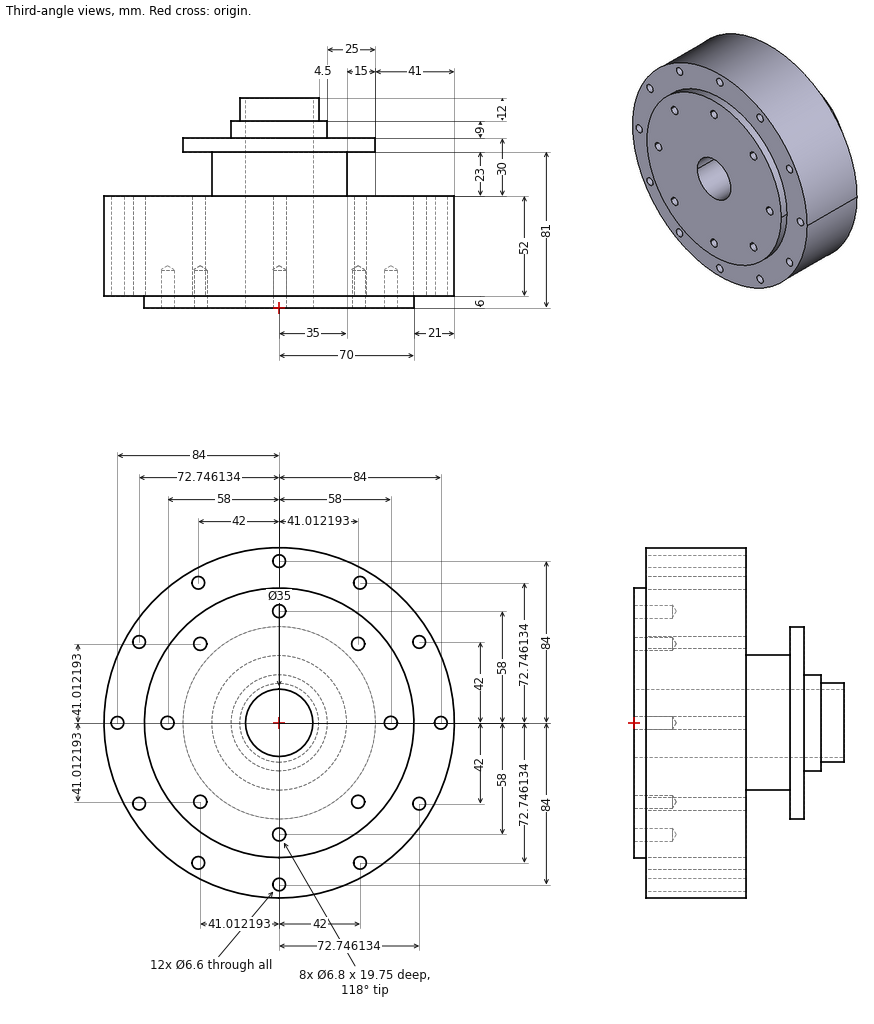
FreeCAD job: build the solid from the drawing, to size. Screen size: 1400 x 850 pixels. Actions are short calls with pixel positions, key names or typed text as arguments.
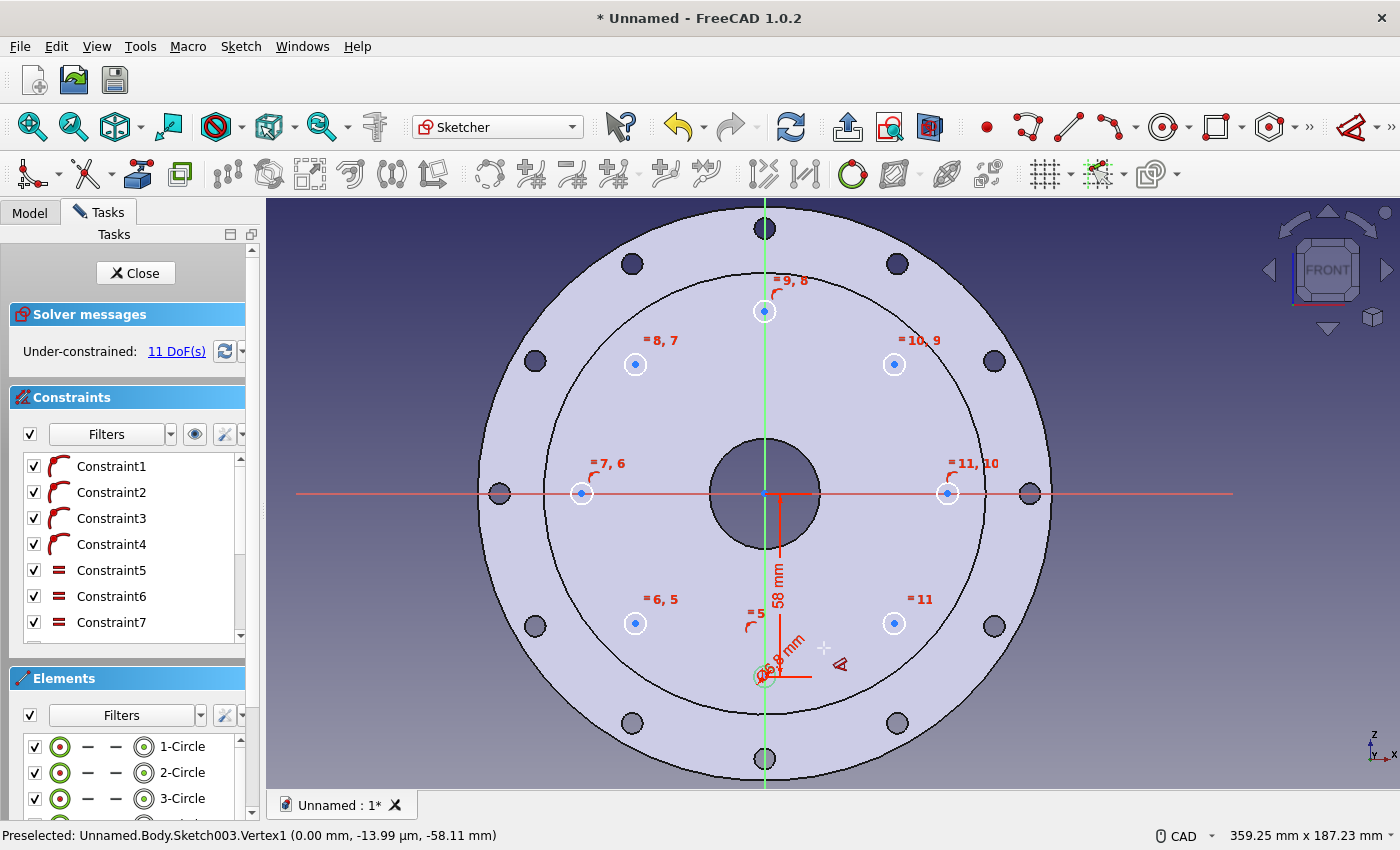
click(582, 494)
click(673, 528)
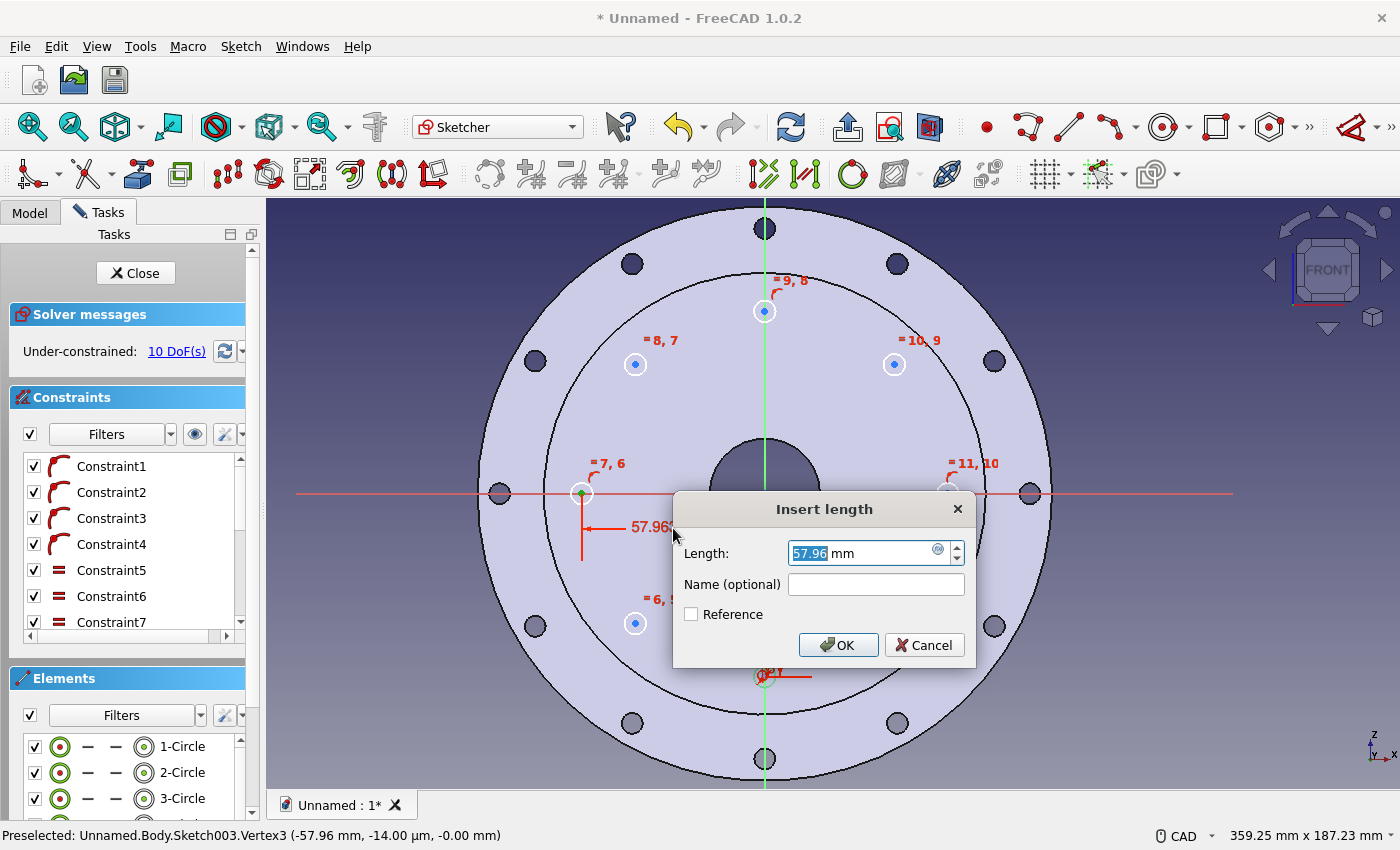
text(58)
key(Return)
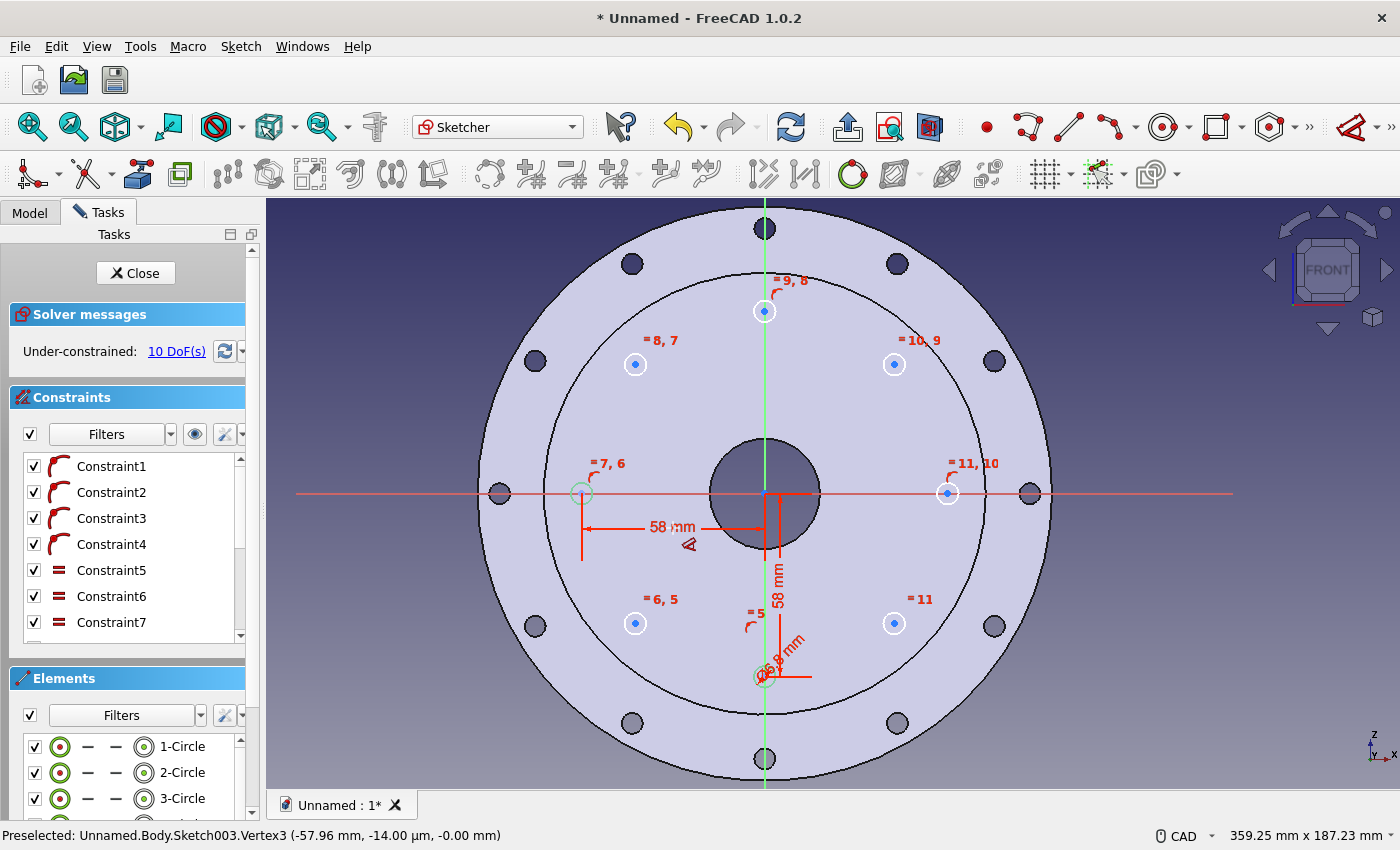
click(765, 311)
click(799, 403)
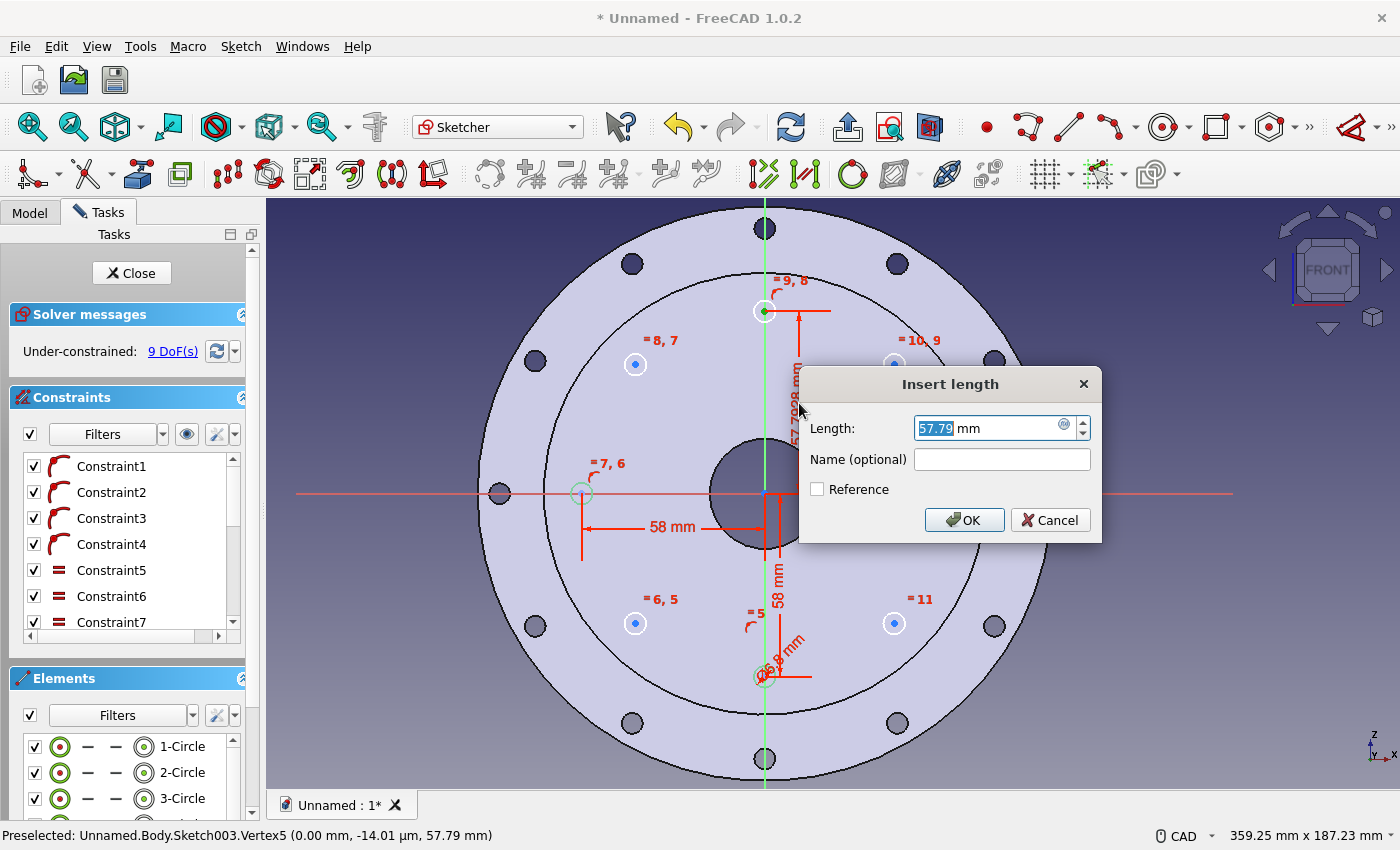
text(58)
key(Return)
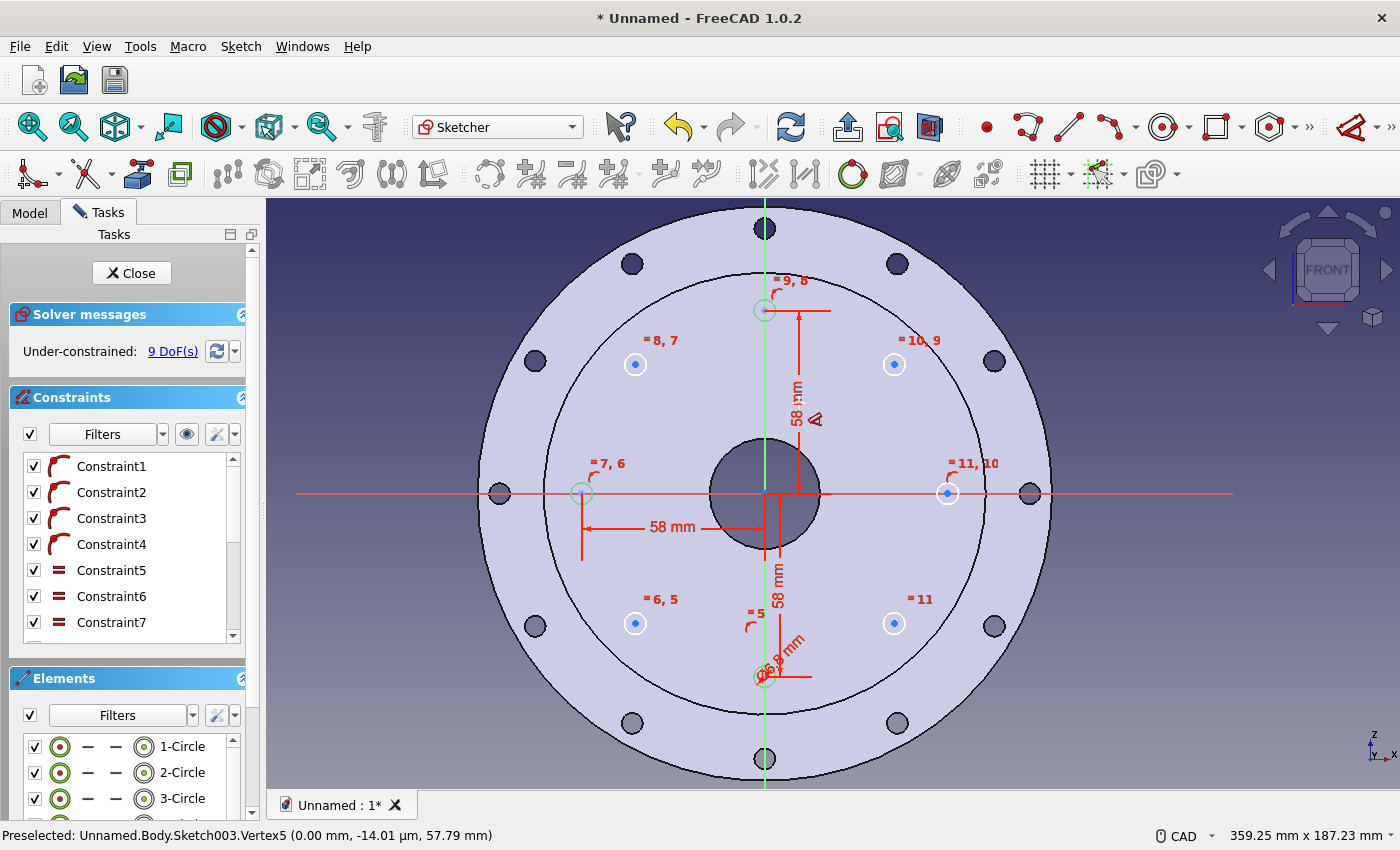
click(948, 494)
click(856, 528)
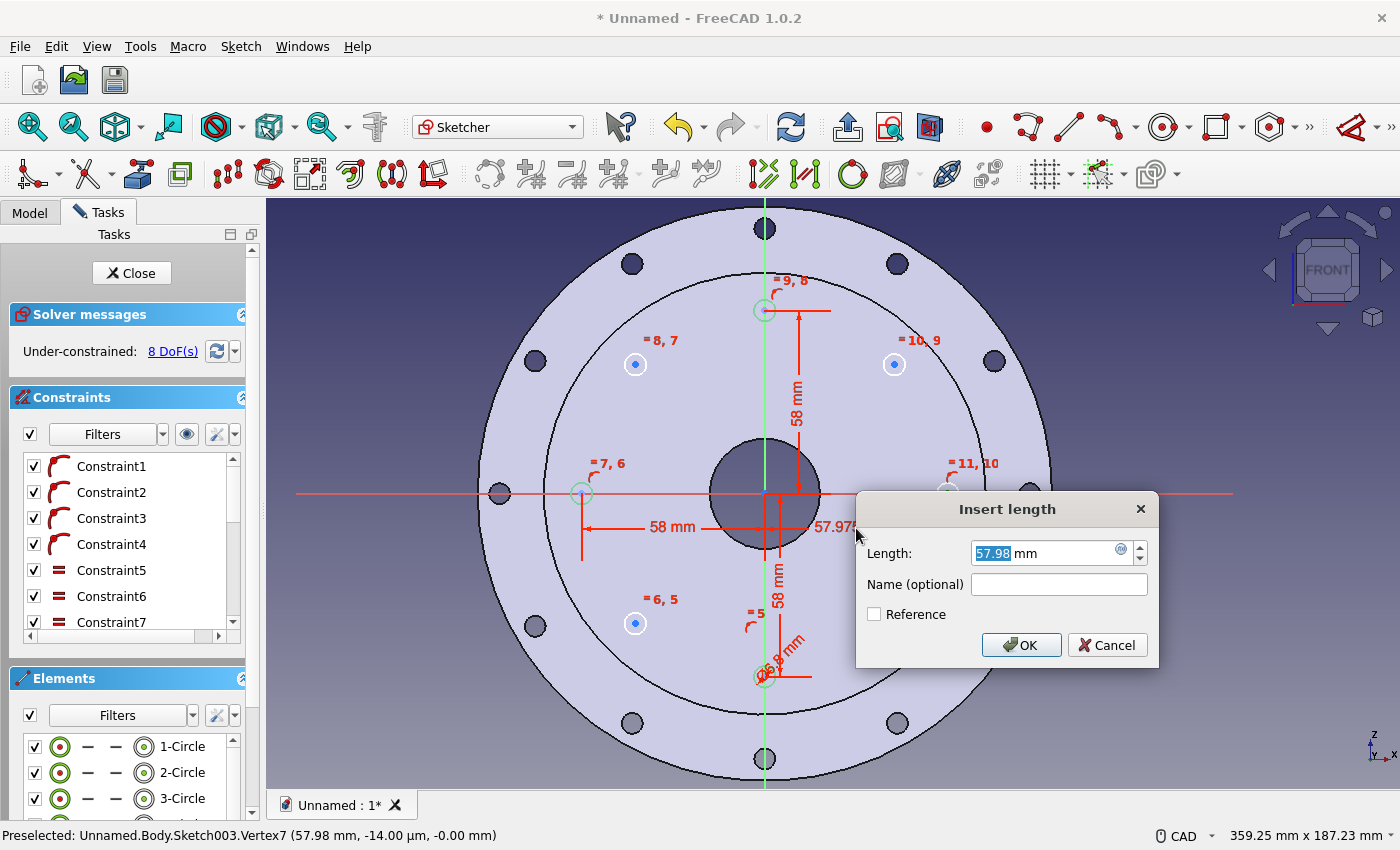
text(58)
key(Return)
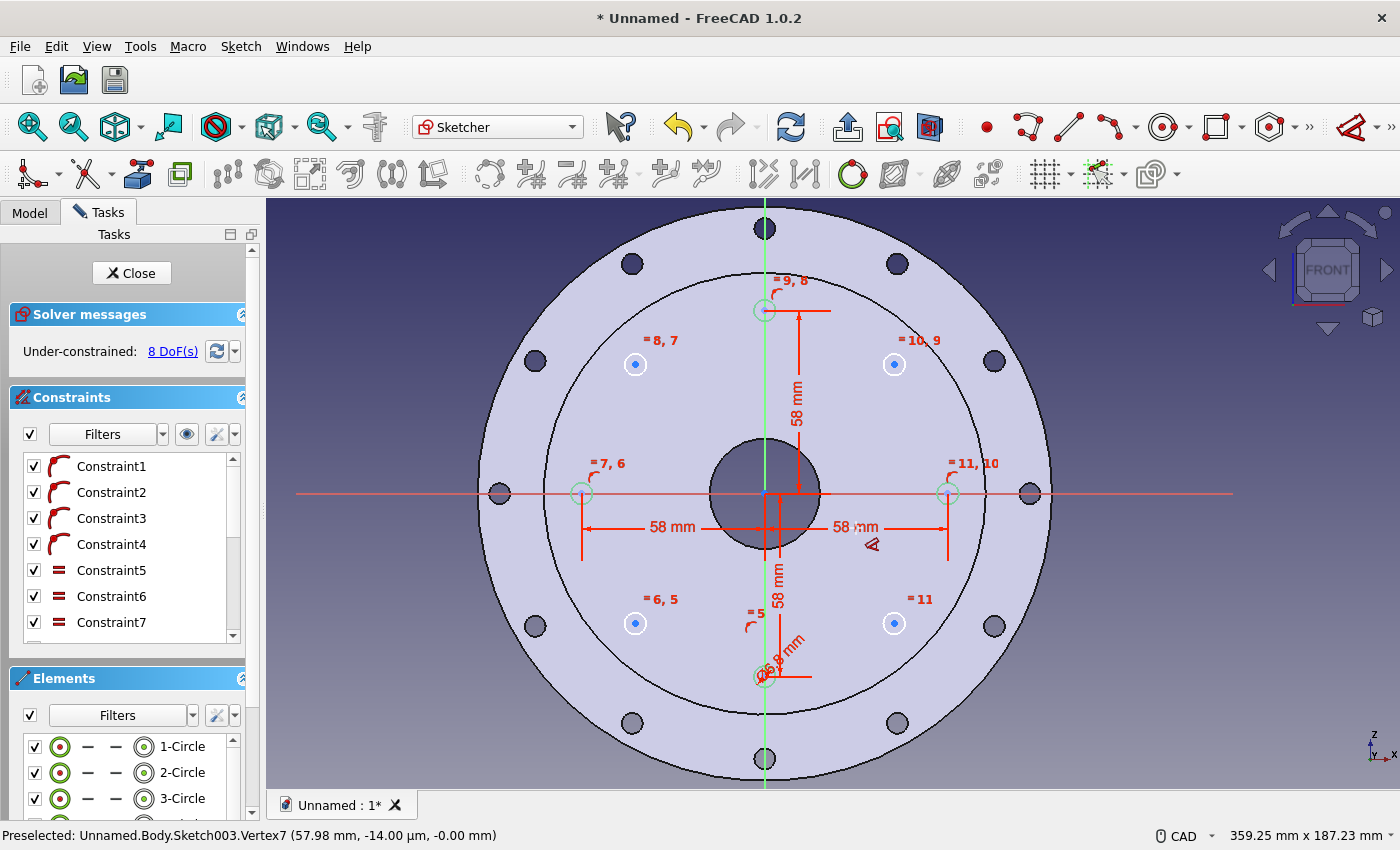
click(635, 624)
click(700, 658)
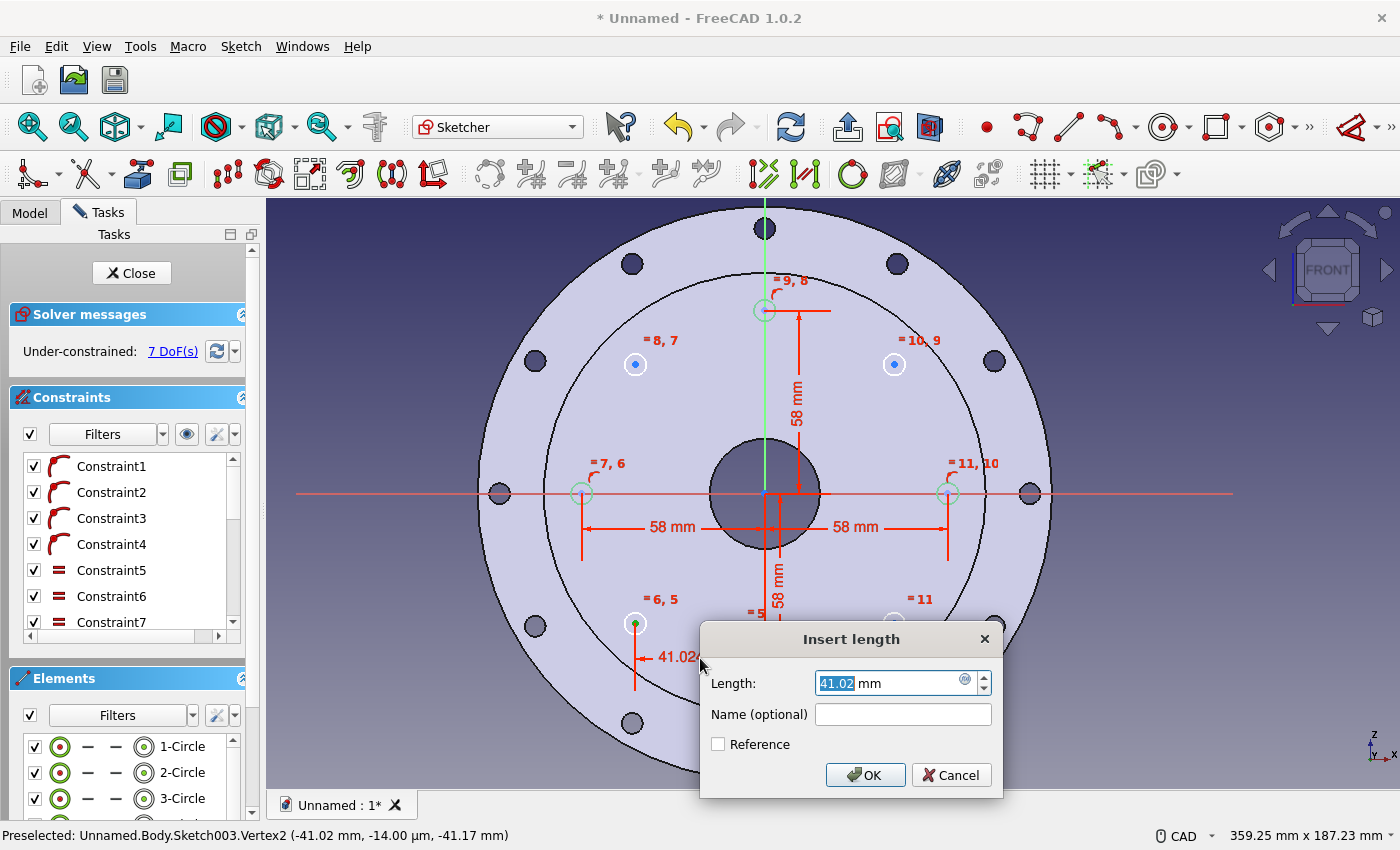
text(41.012193)
key(Return)